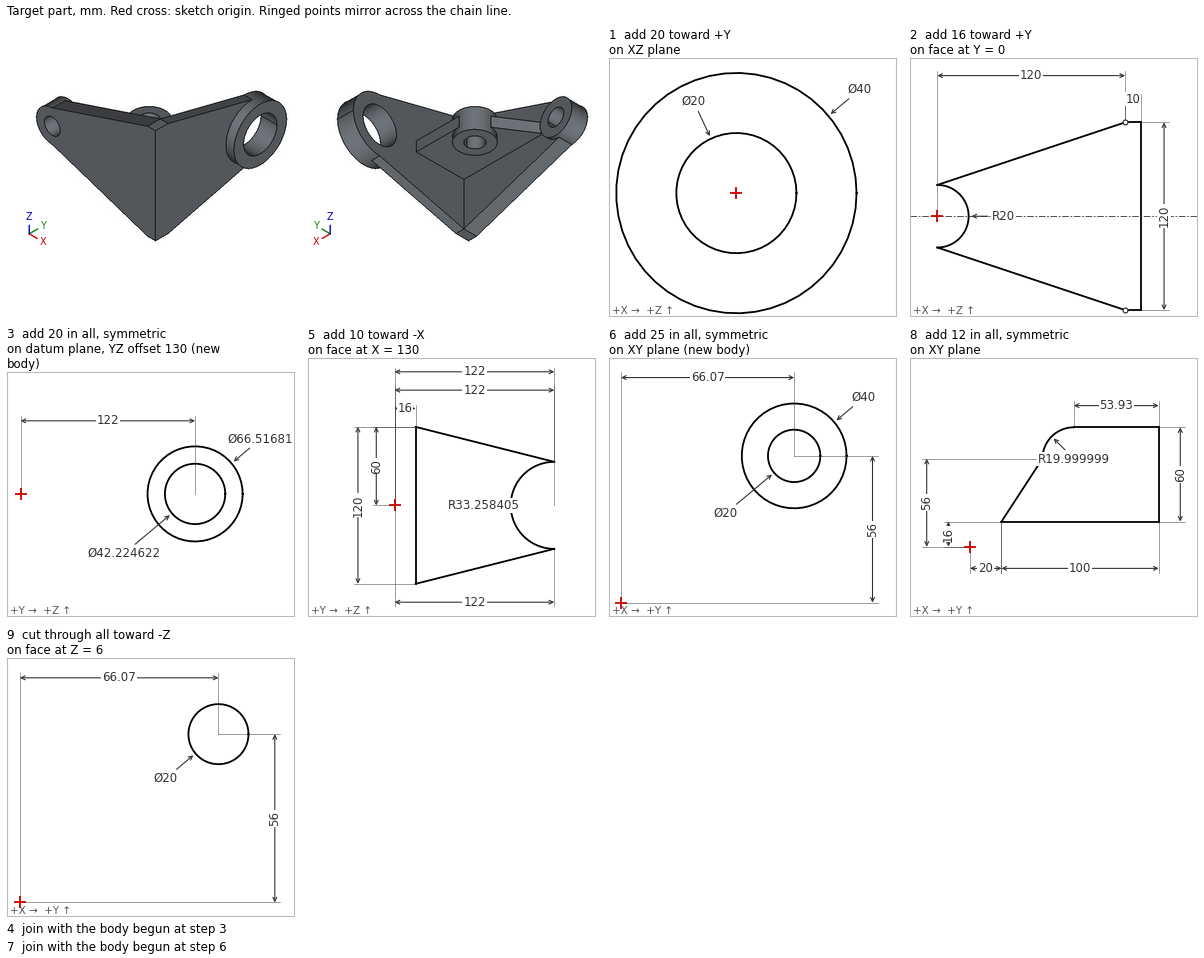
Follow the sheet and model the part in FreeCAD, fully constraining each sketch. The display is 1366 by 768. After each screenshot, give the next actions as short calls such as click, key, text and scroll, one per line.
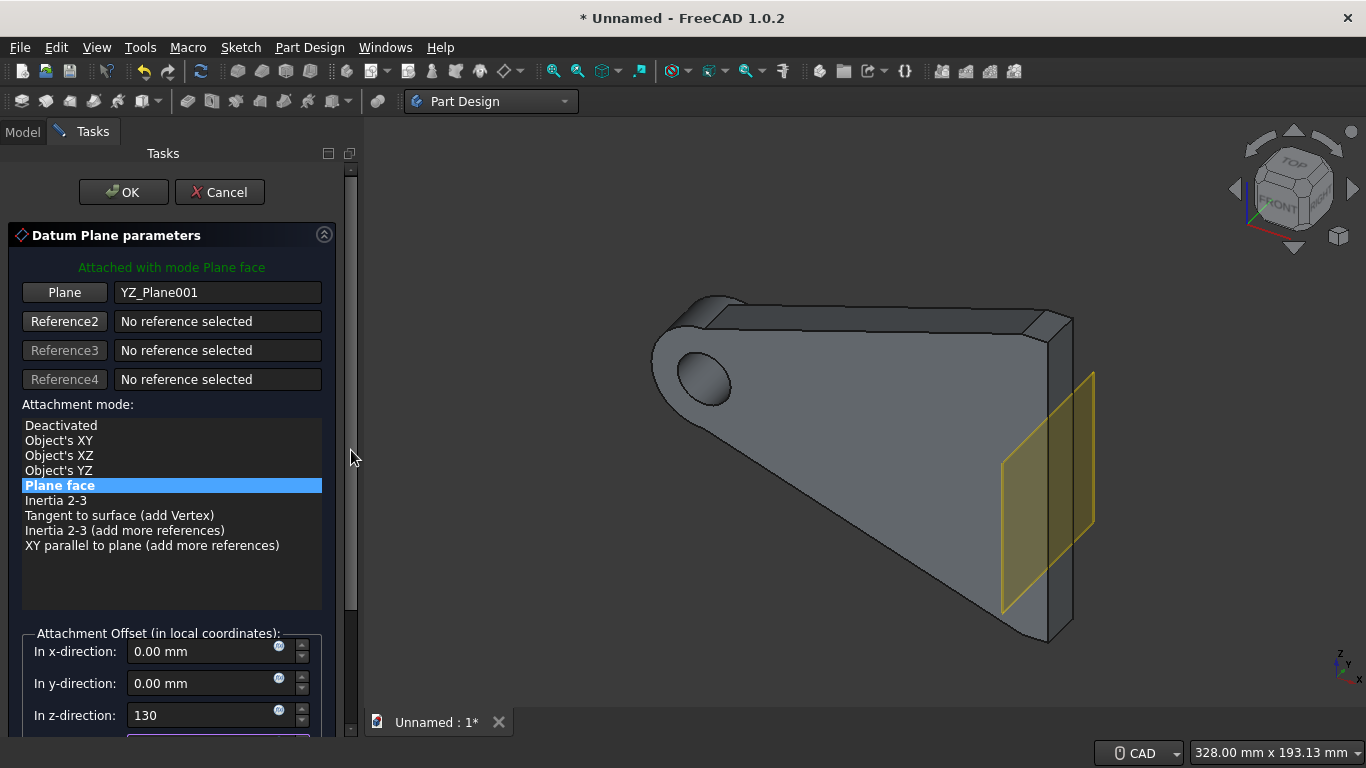
click(124, 192)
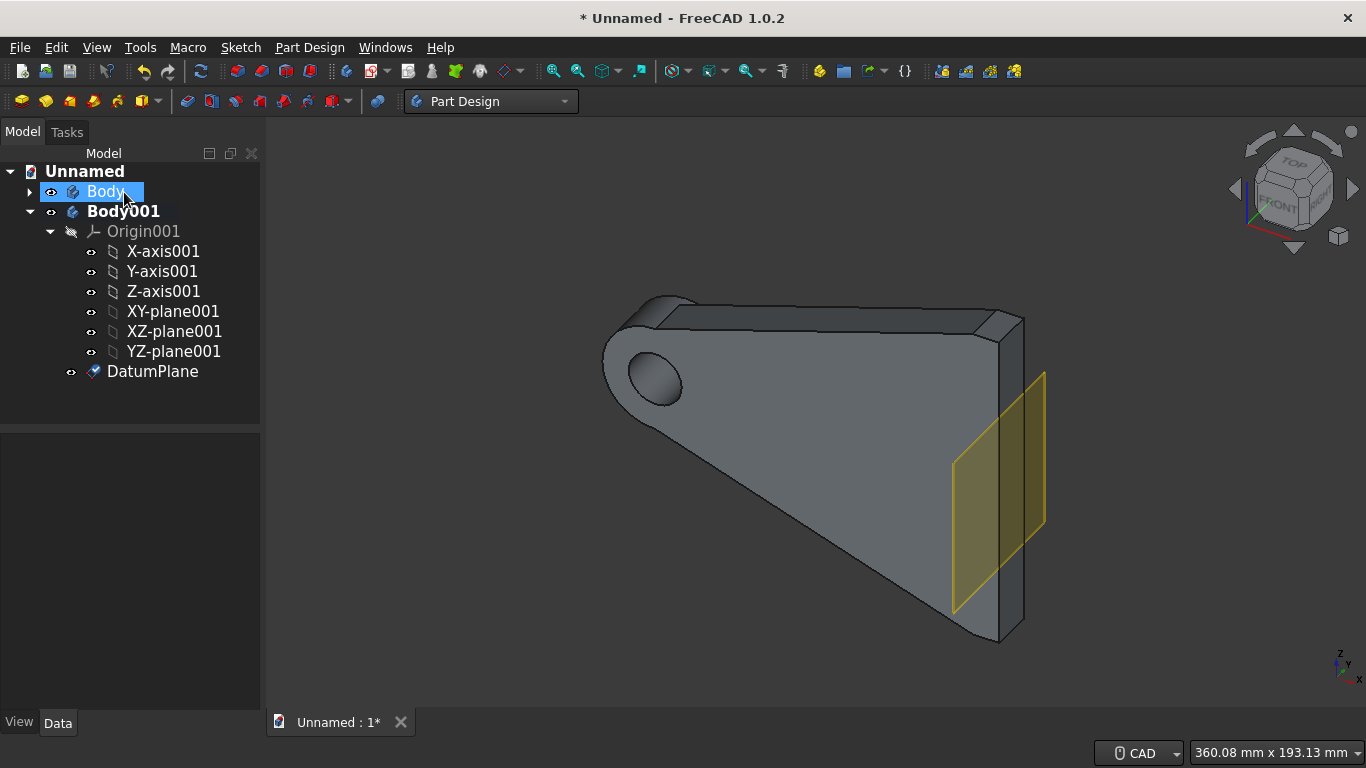
click(116, 372)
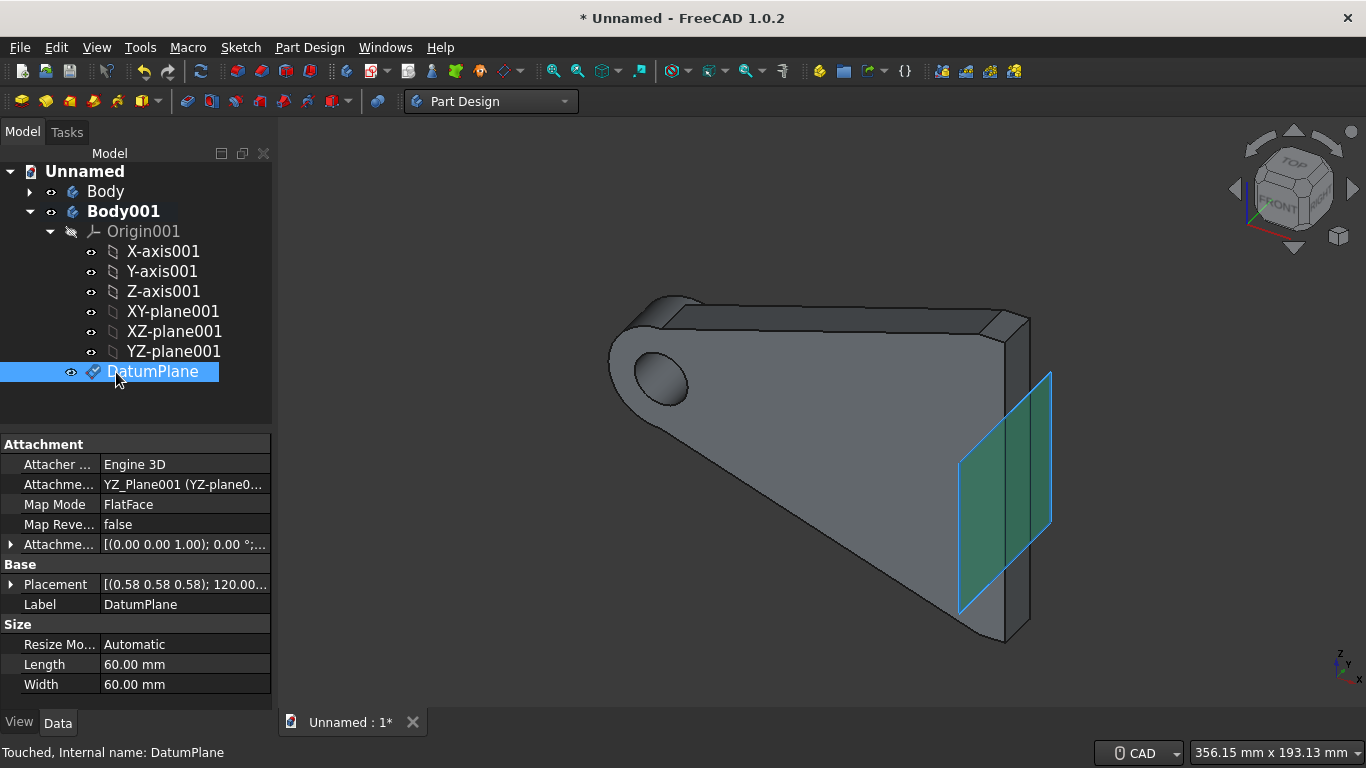
click(372, 72)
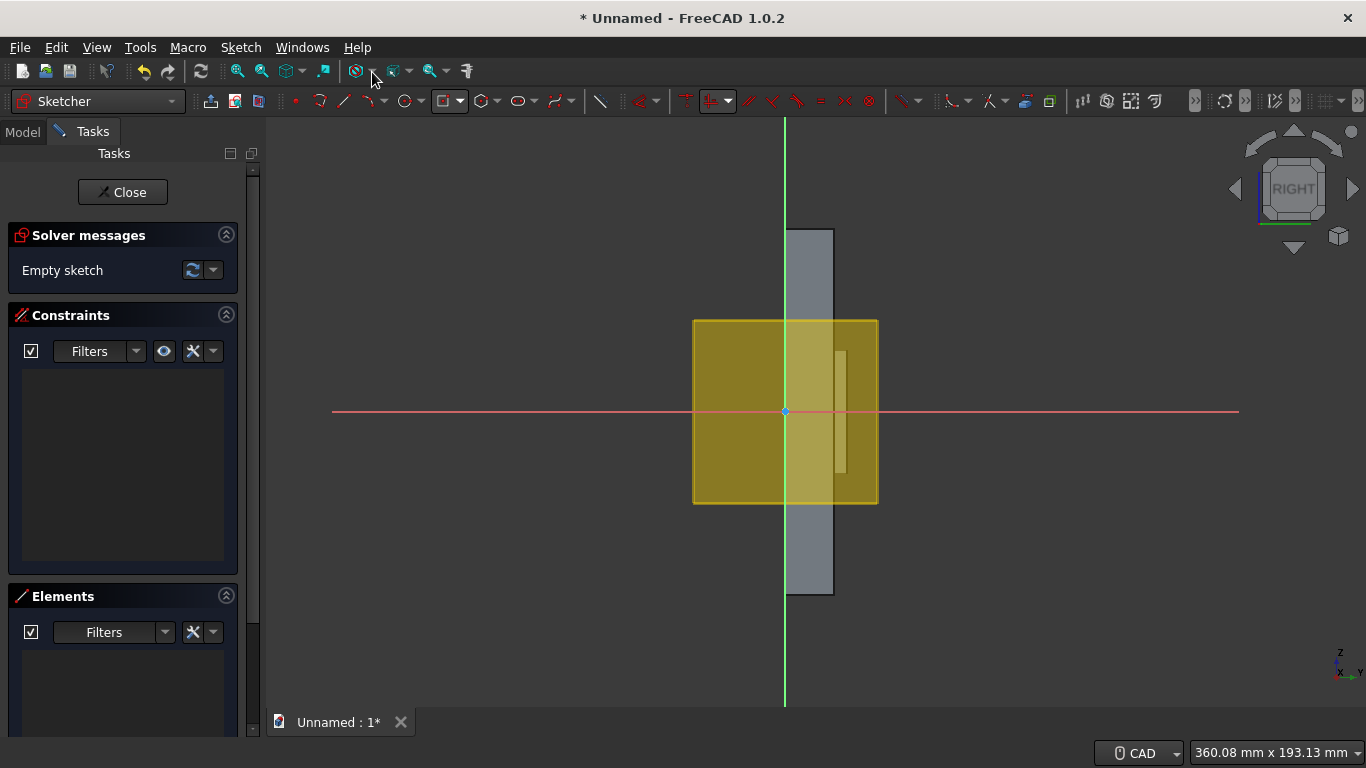
scroll(294, 412, down, 1)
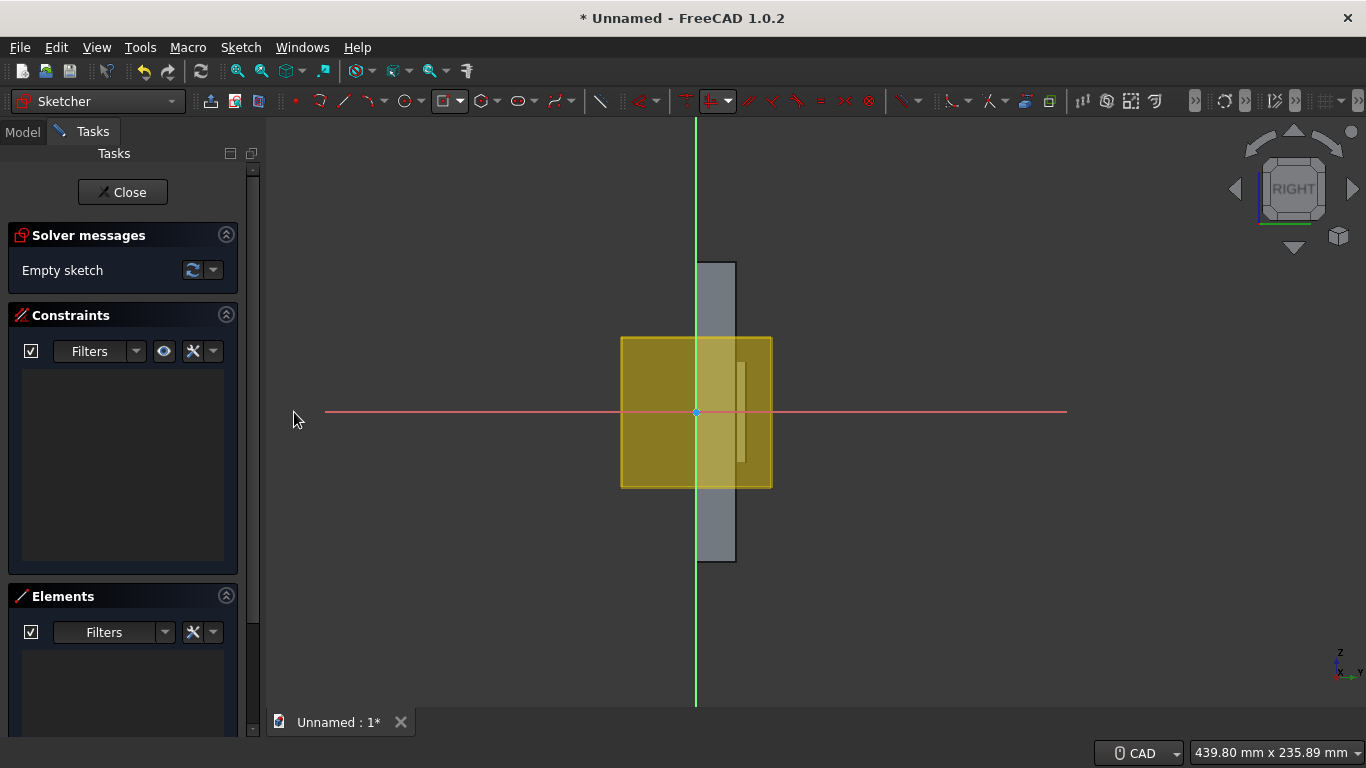
scroll(1181, 412, up, 2)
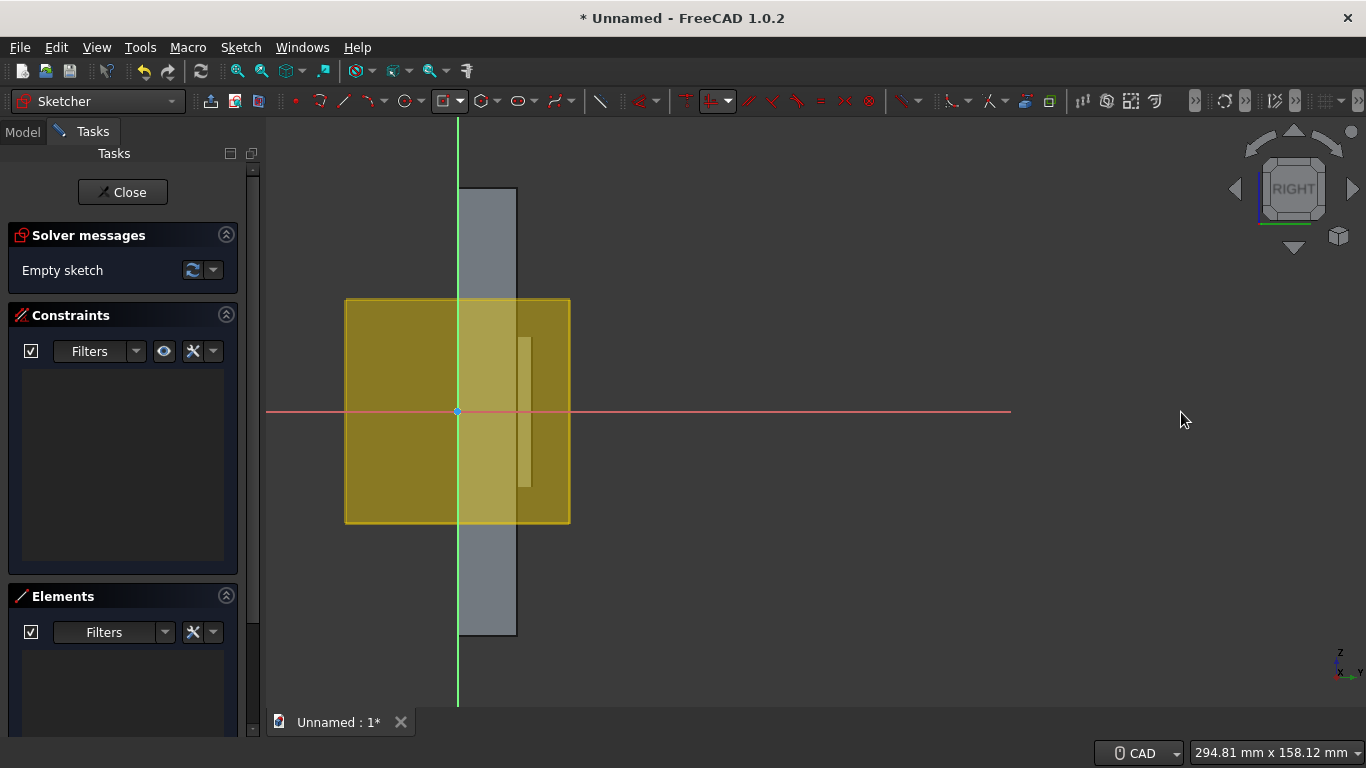
key(g)
key(c)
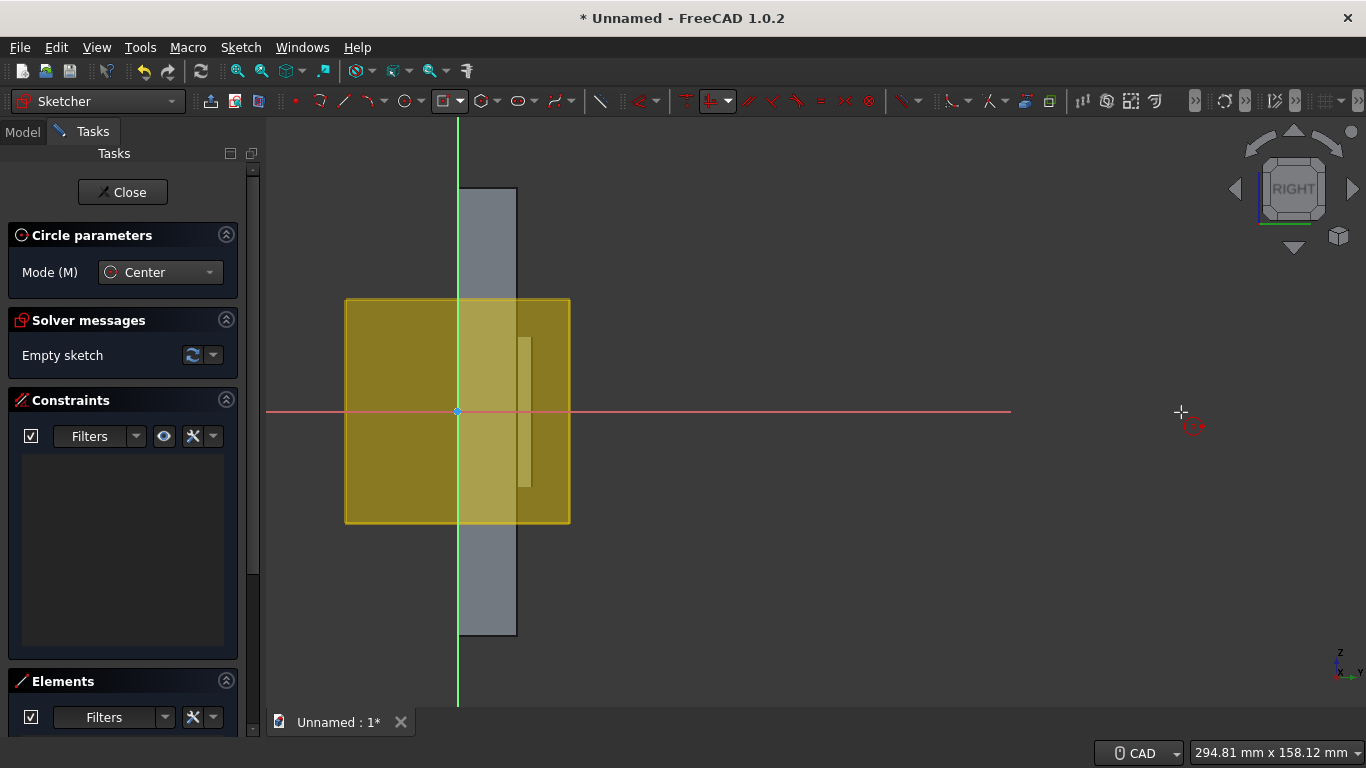
click(913, 412)
click(1001, 324)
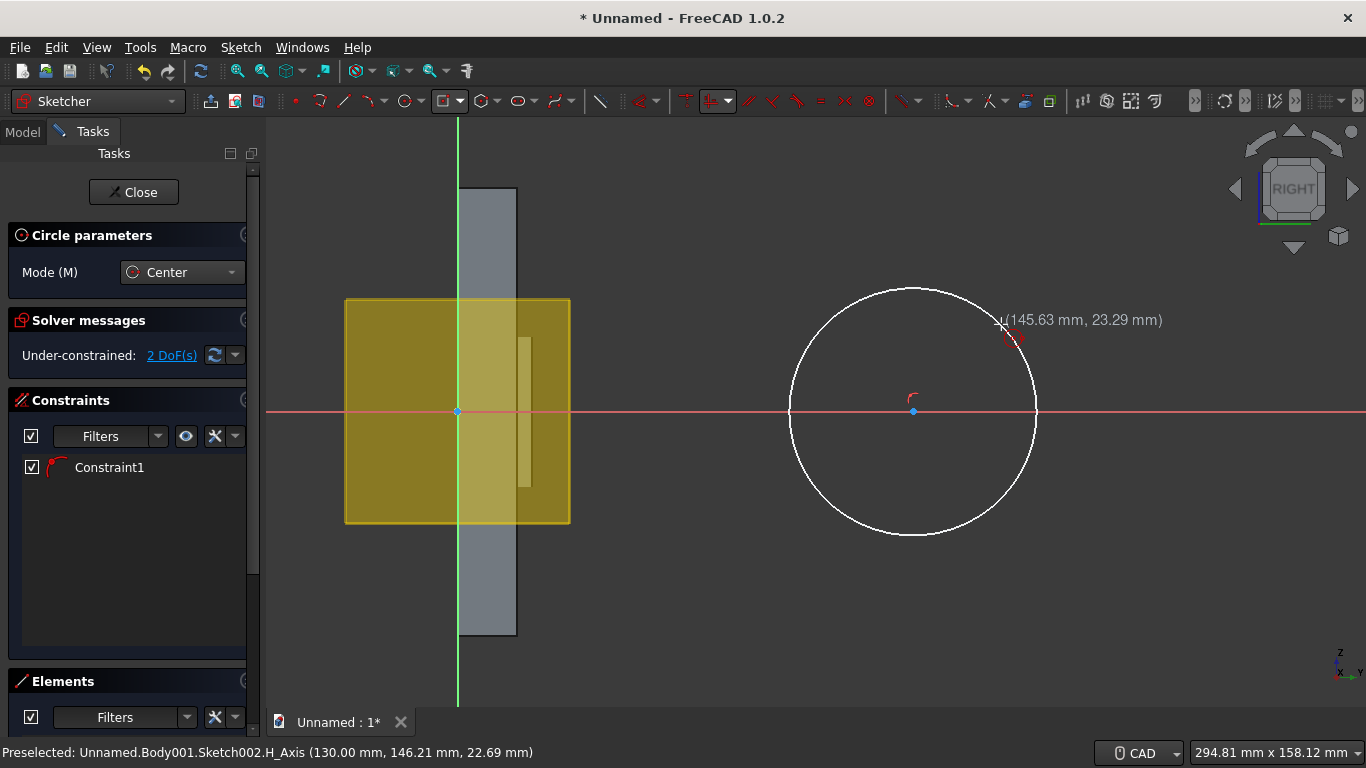
click(913, 412)
click(969, 356)
key(Escape)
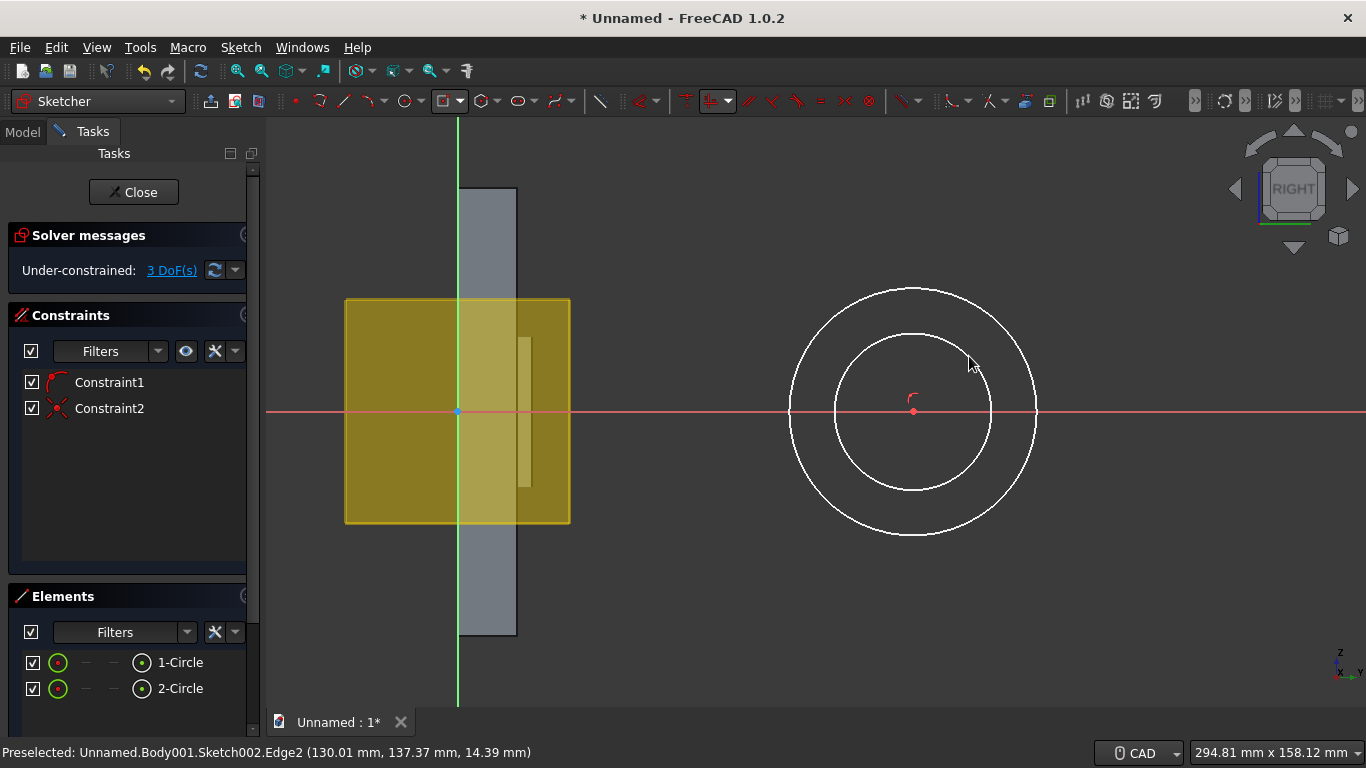
click(640, 102)